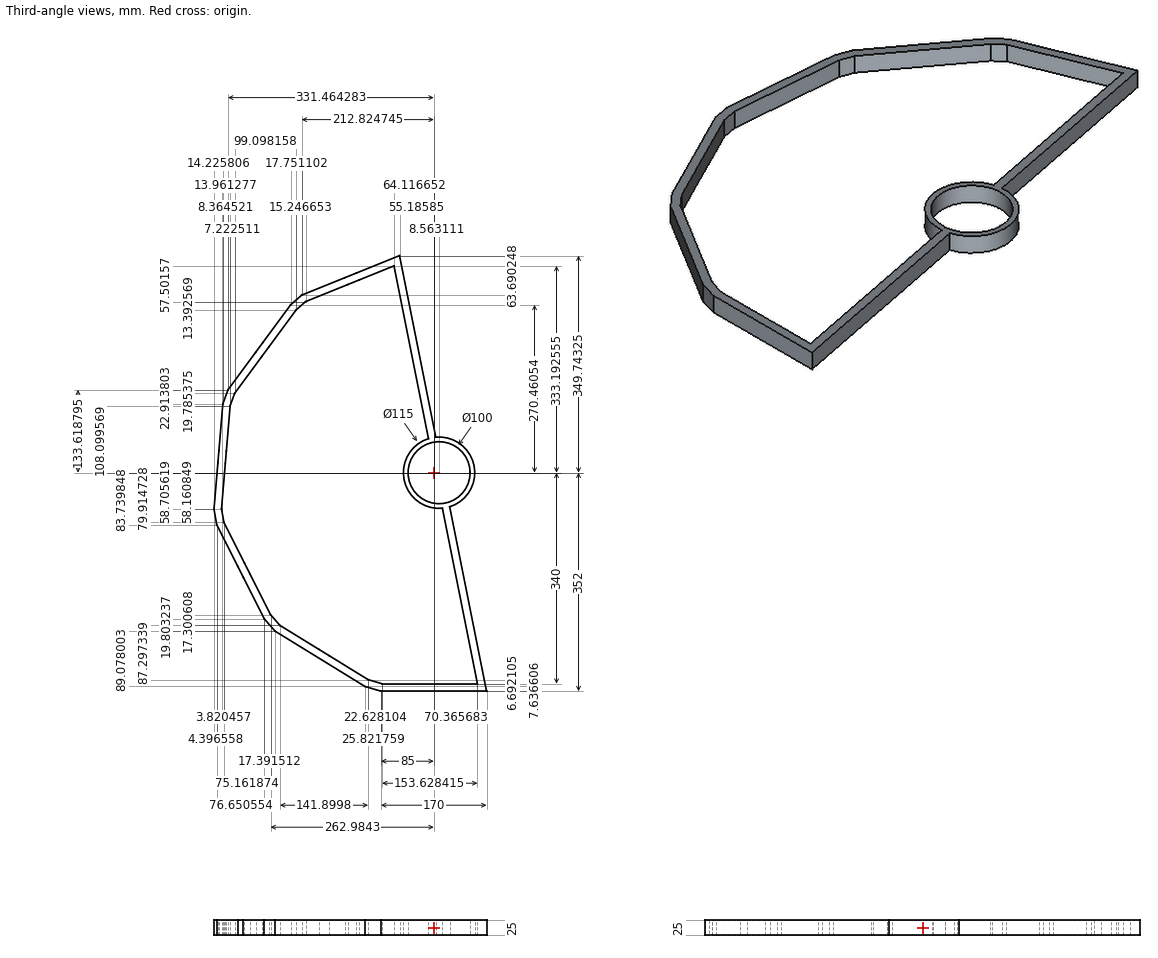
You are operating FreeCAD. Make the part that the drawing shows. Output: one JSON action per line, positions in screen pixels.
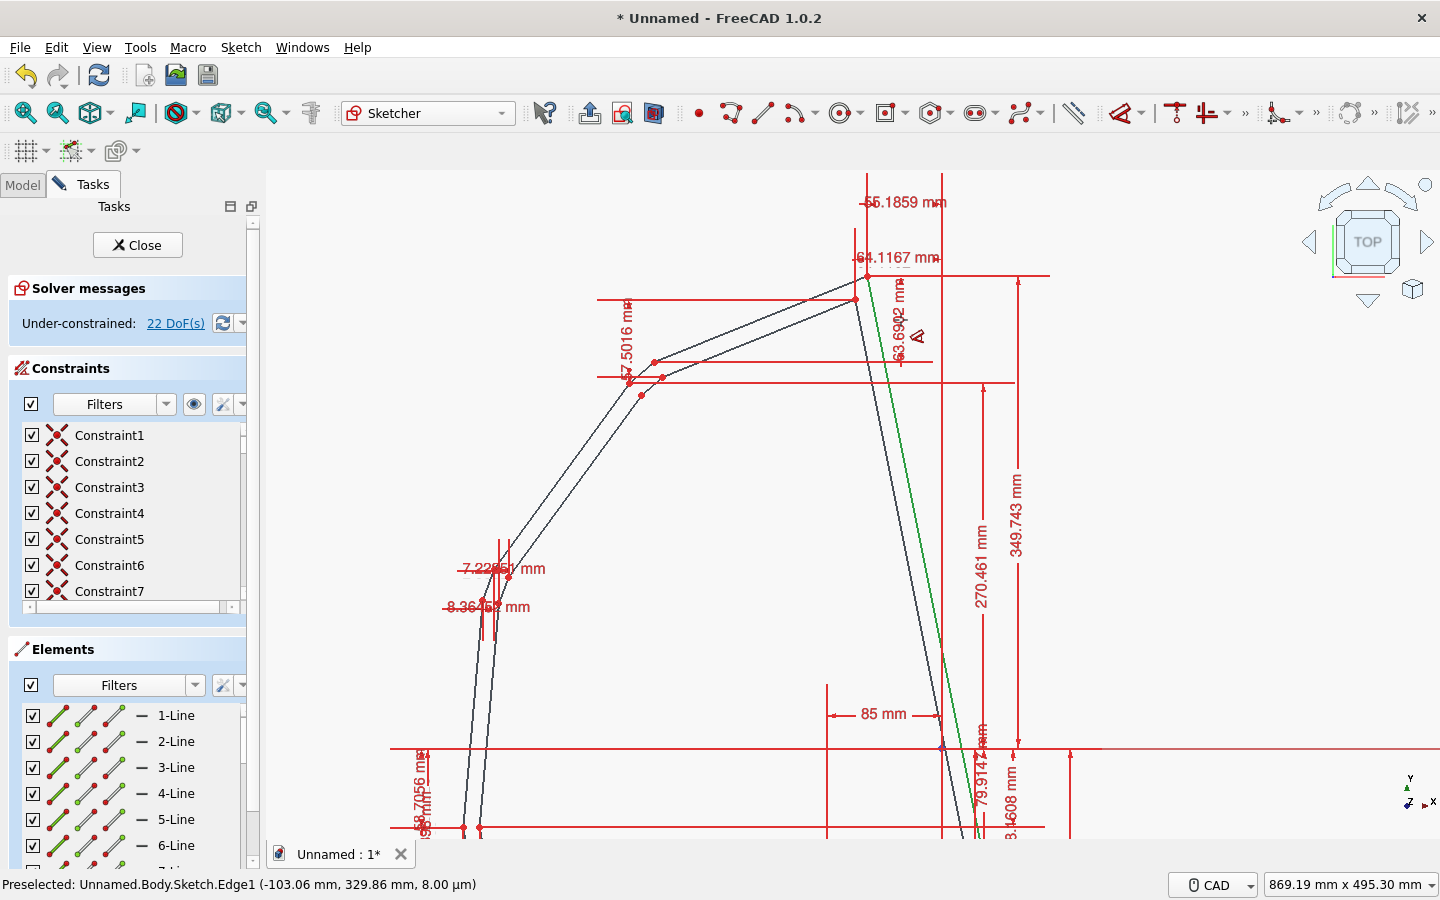
{"action": "scroll", "coordinate": [647, 369], "scroll_direction": "up", "scroll_amount": 3}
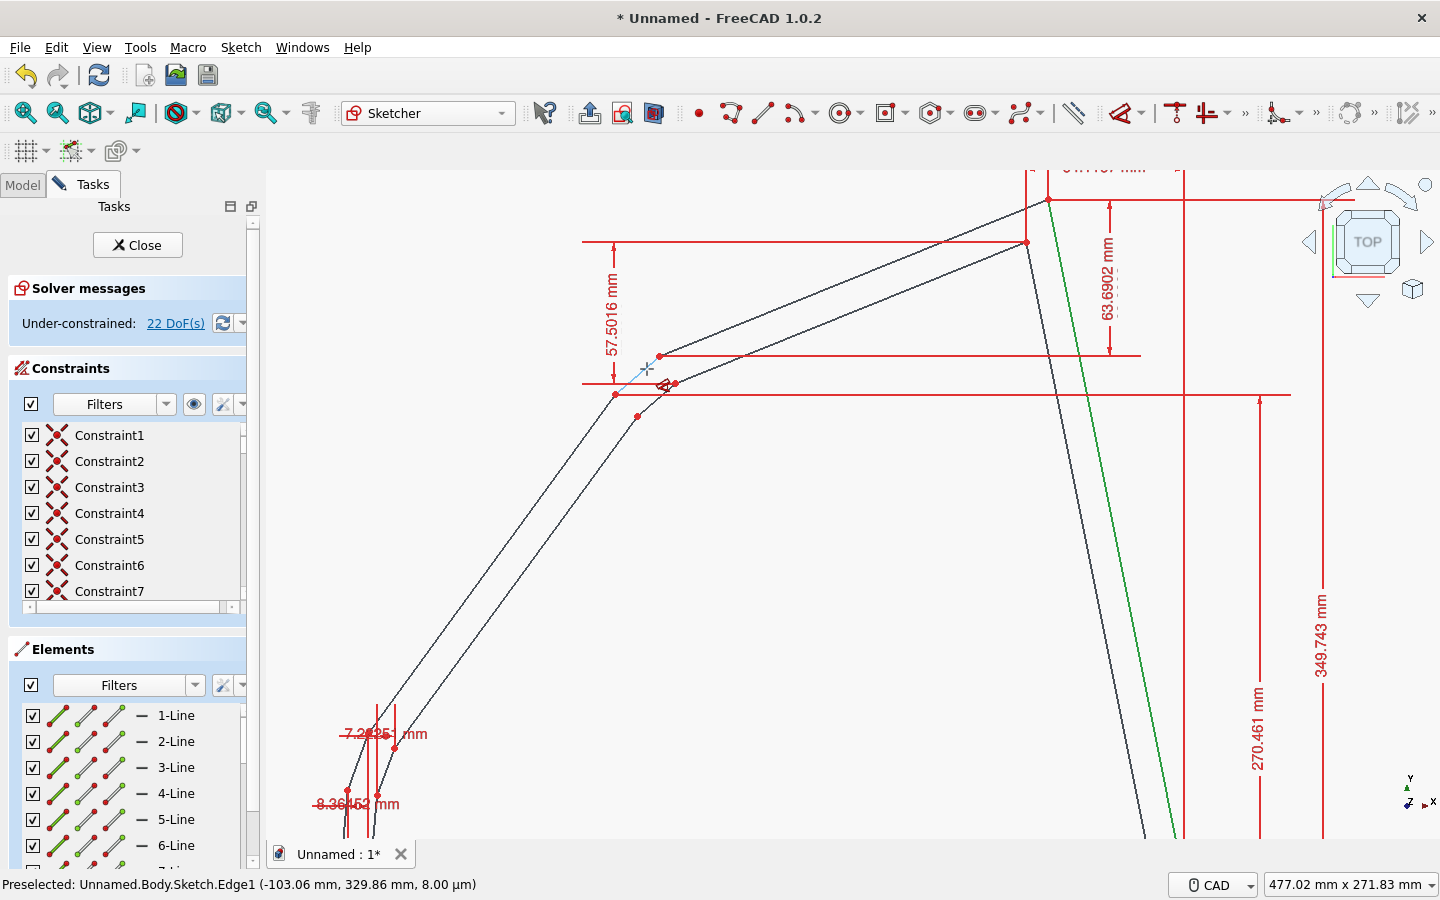
{"action": "left_click", "coordinate": [647, 368]}
{"action": "left_click", "coordinate": [648, 429]}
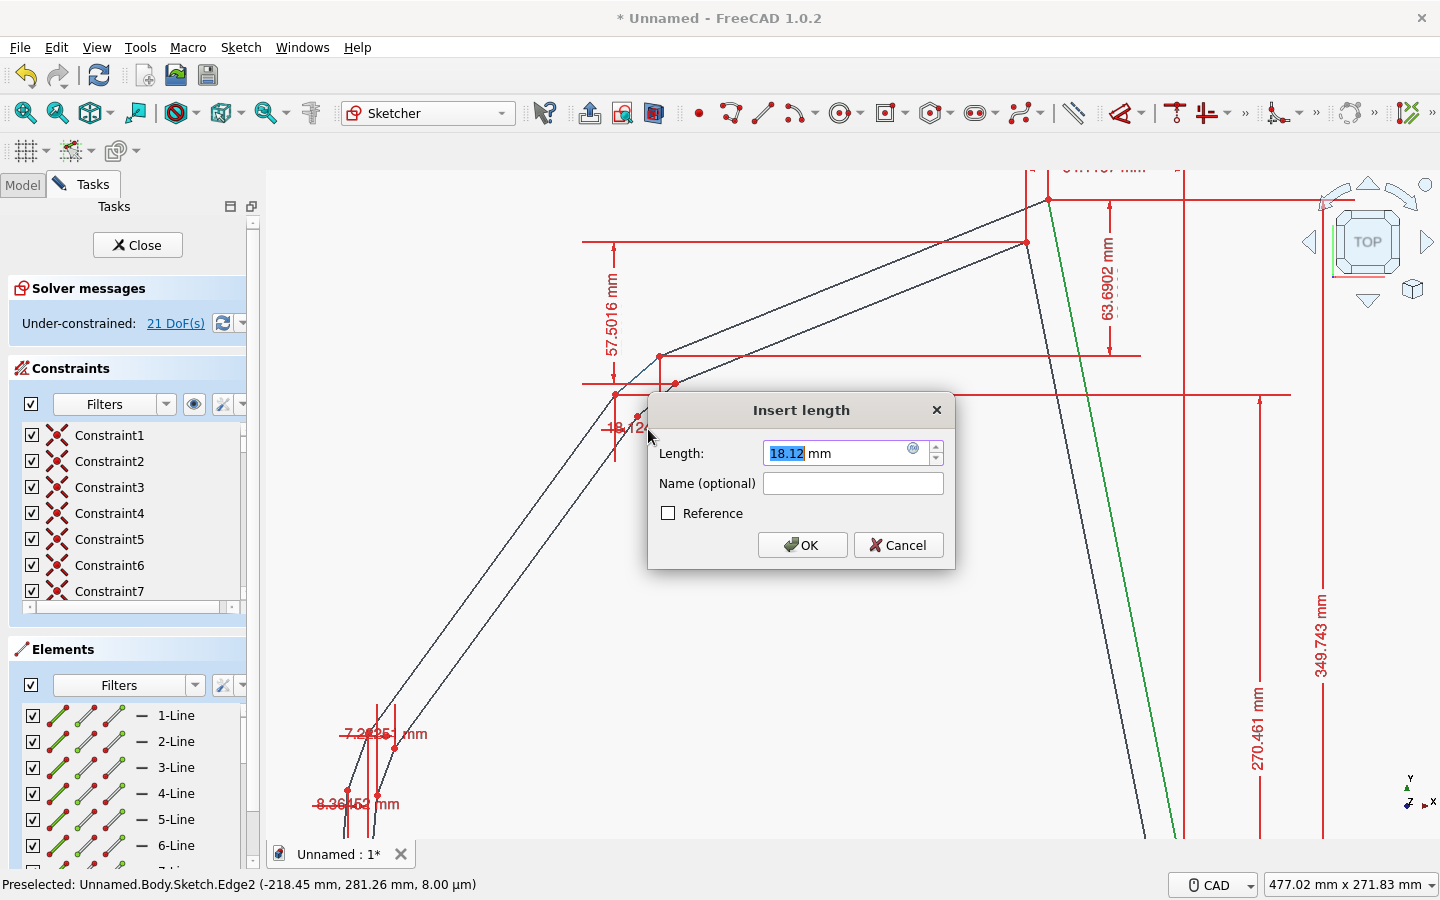
{"action": "type", "text": "17.751102"}
{"action": "key", "text": "Return"}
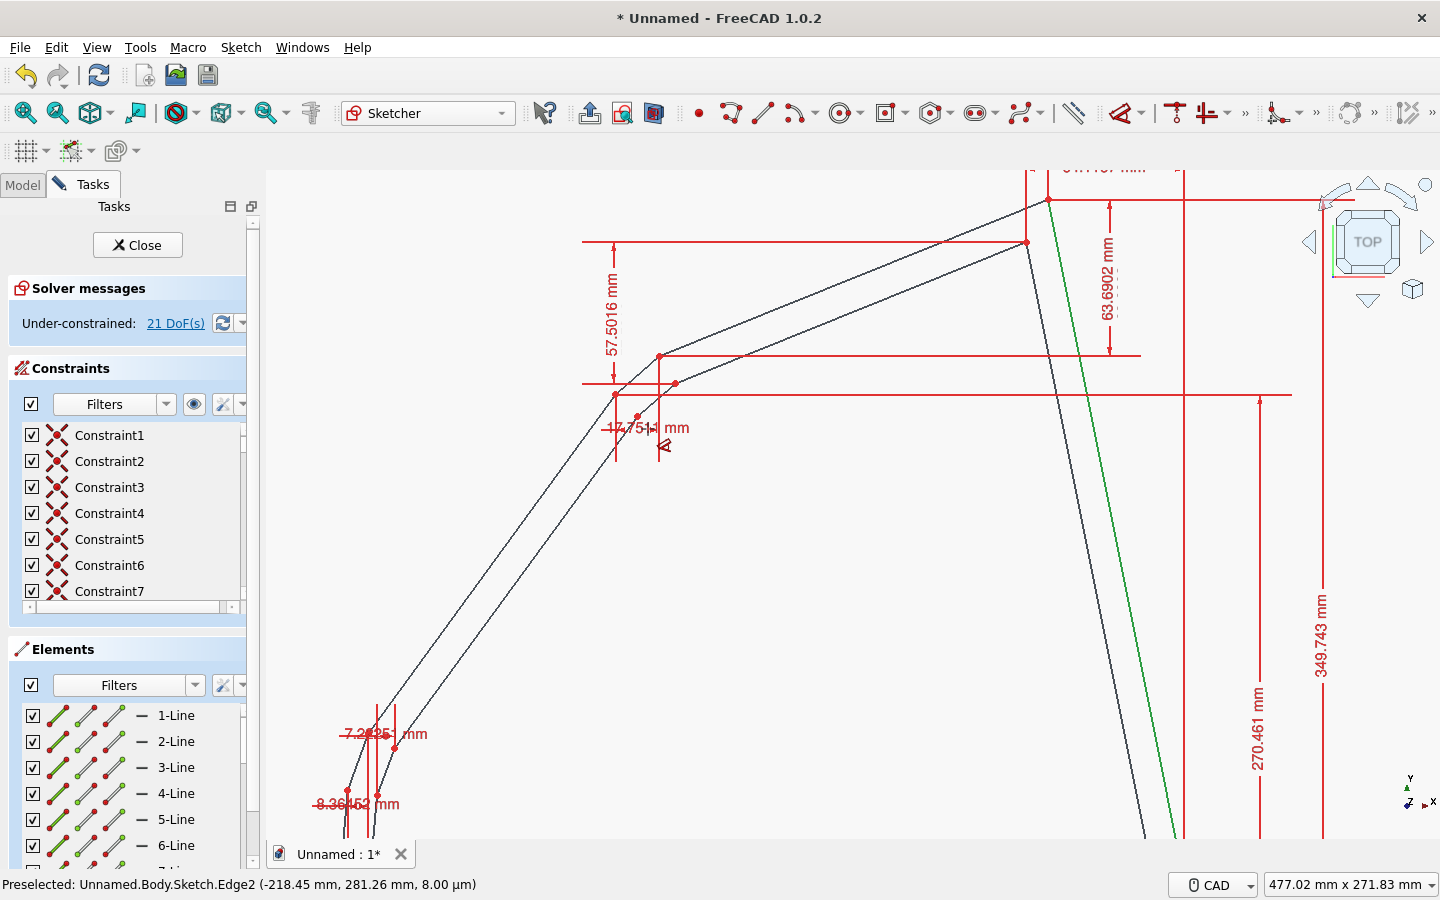
{"action": "left_click", "coordinate": [362, 751]}
{"action": "left_click", "coordinate": [314, 762]}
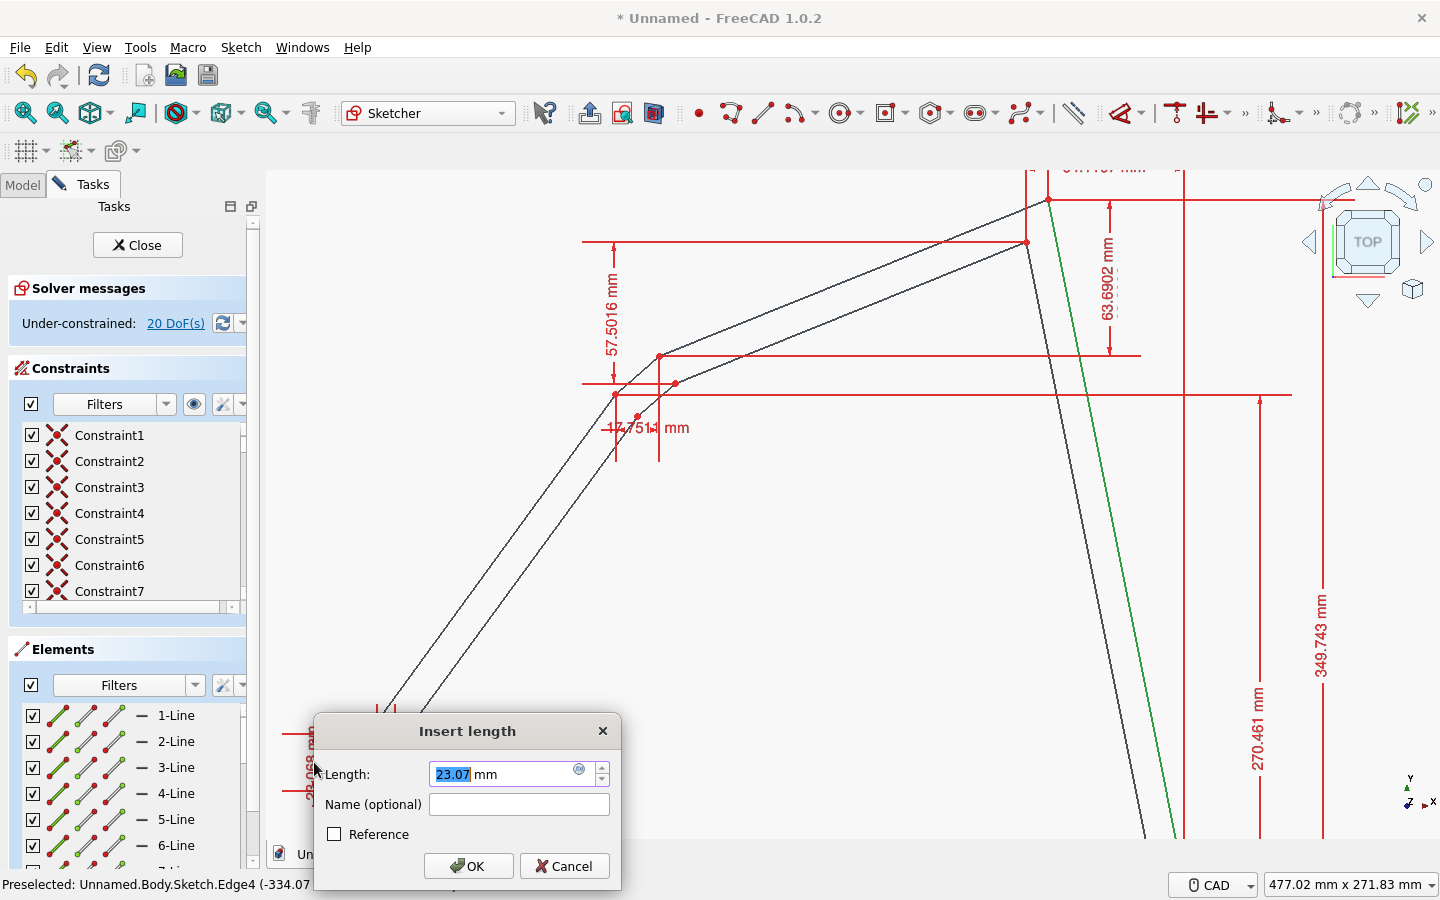
{"action": "type", "text": "22.913803"}
{"action": "key", "text": "Return"}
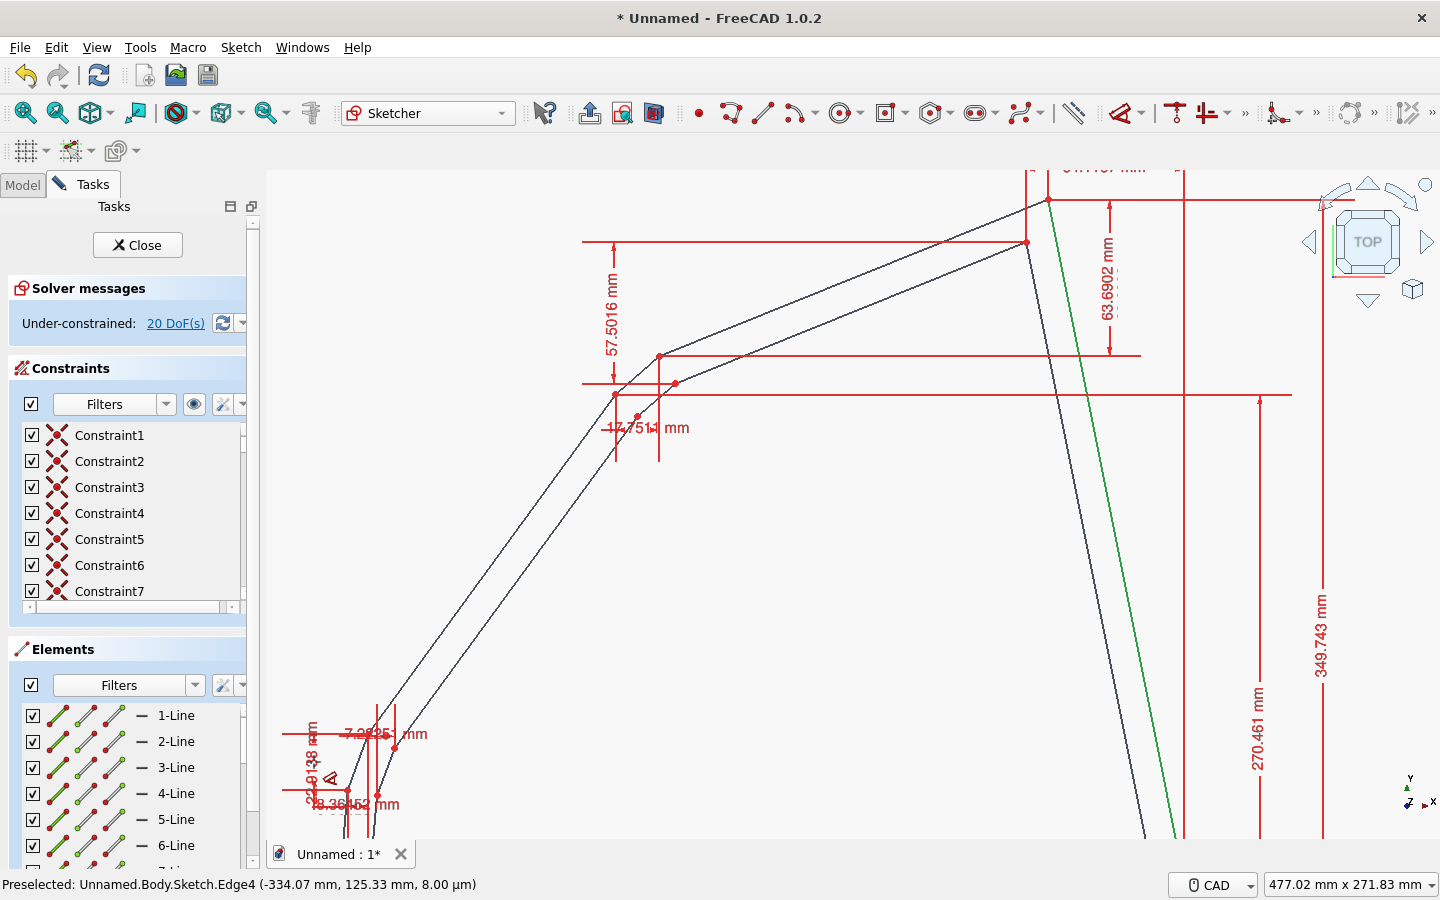
{"action": "scroll", "coordinate": [762, 322], "scroll_direction": "down", "scroll_amount": 7}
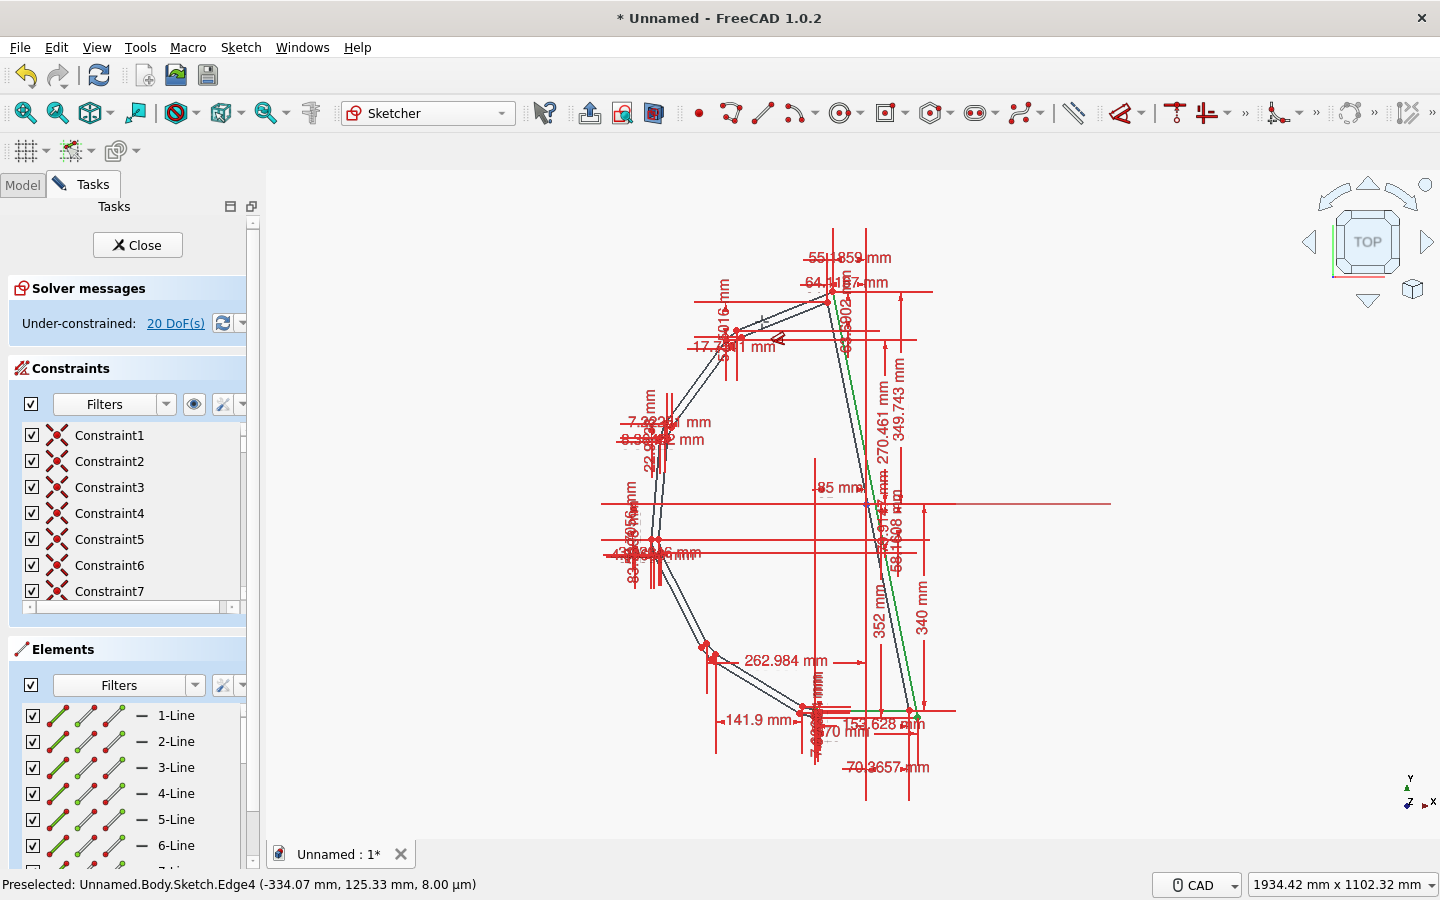
{"action": "scroll", "coordinate": [658, 468], "scroll_direction": "up", "scroll_amount": 8}